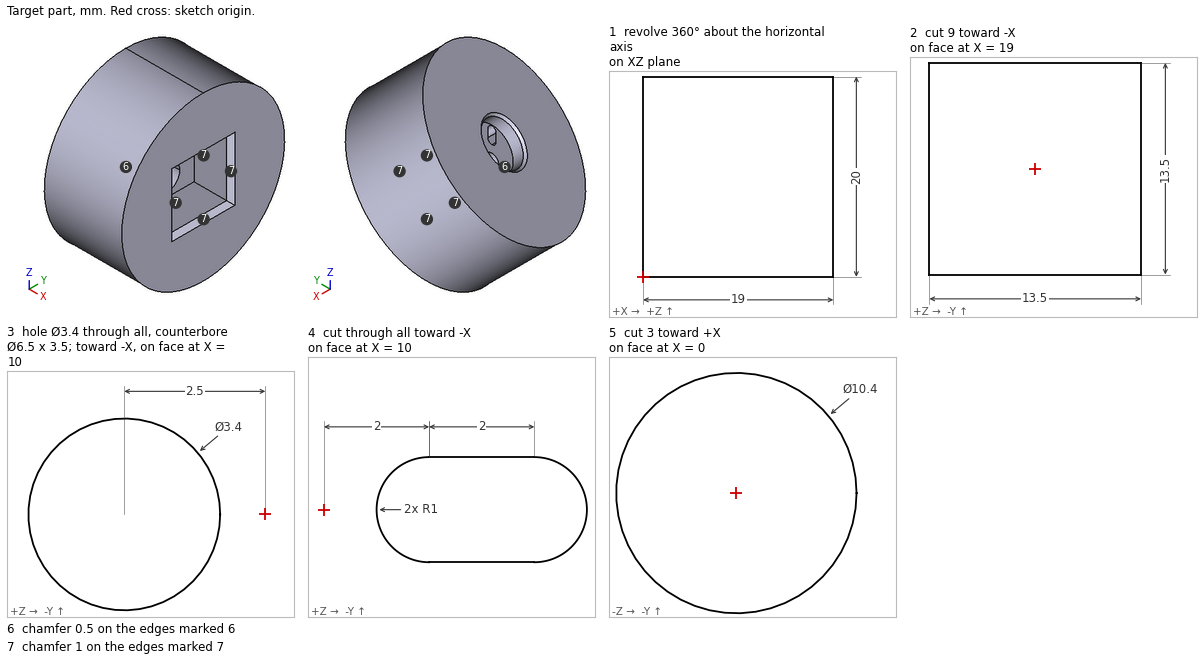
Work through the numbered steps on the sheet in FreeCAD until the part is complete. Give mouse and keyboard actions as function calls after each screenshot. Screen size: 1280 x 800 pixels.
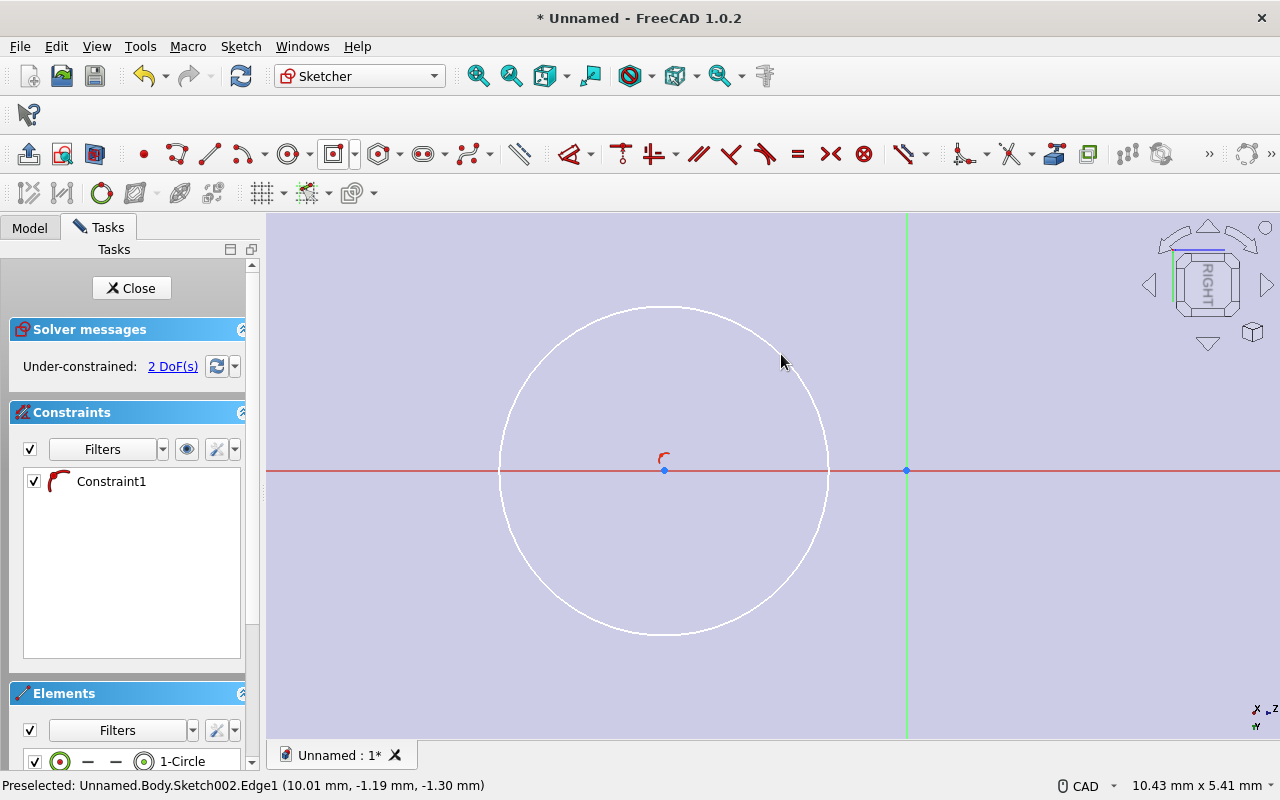
click(568, 154)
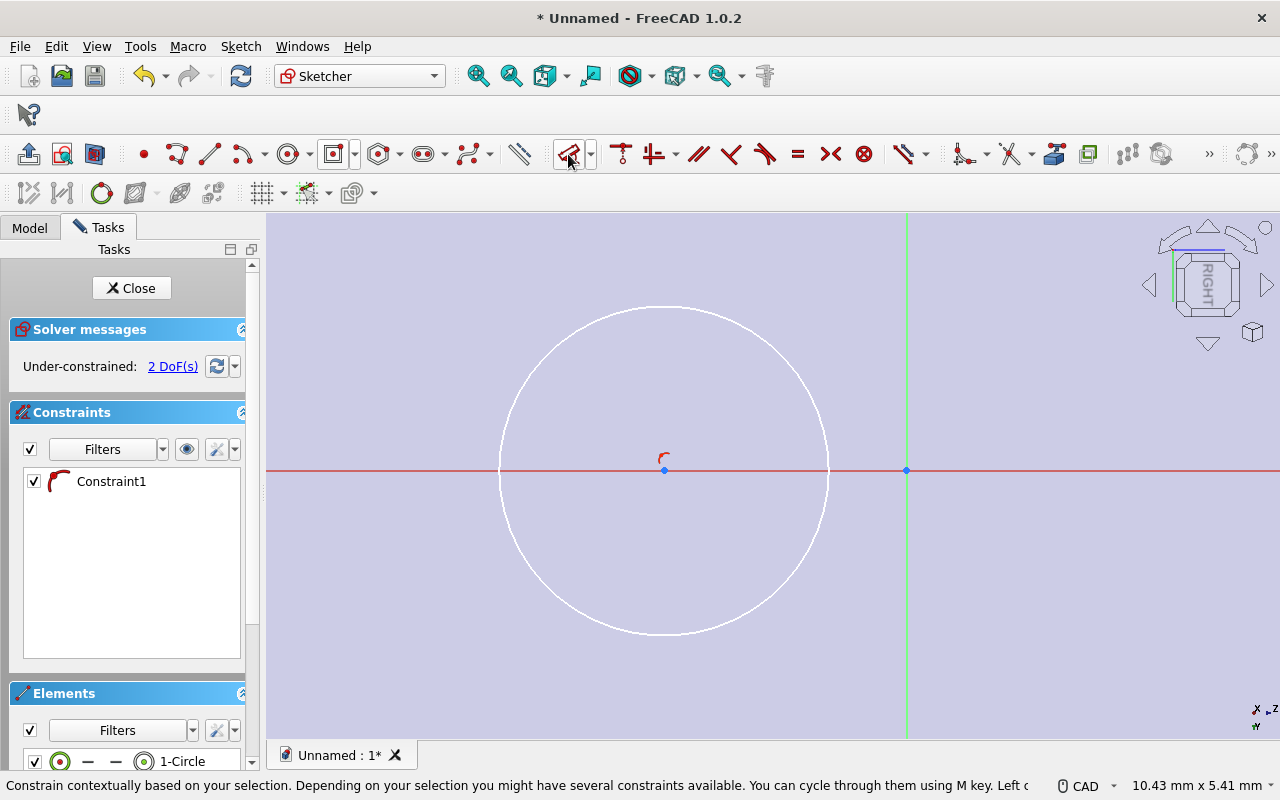
click(780, 354)
click(803, 331)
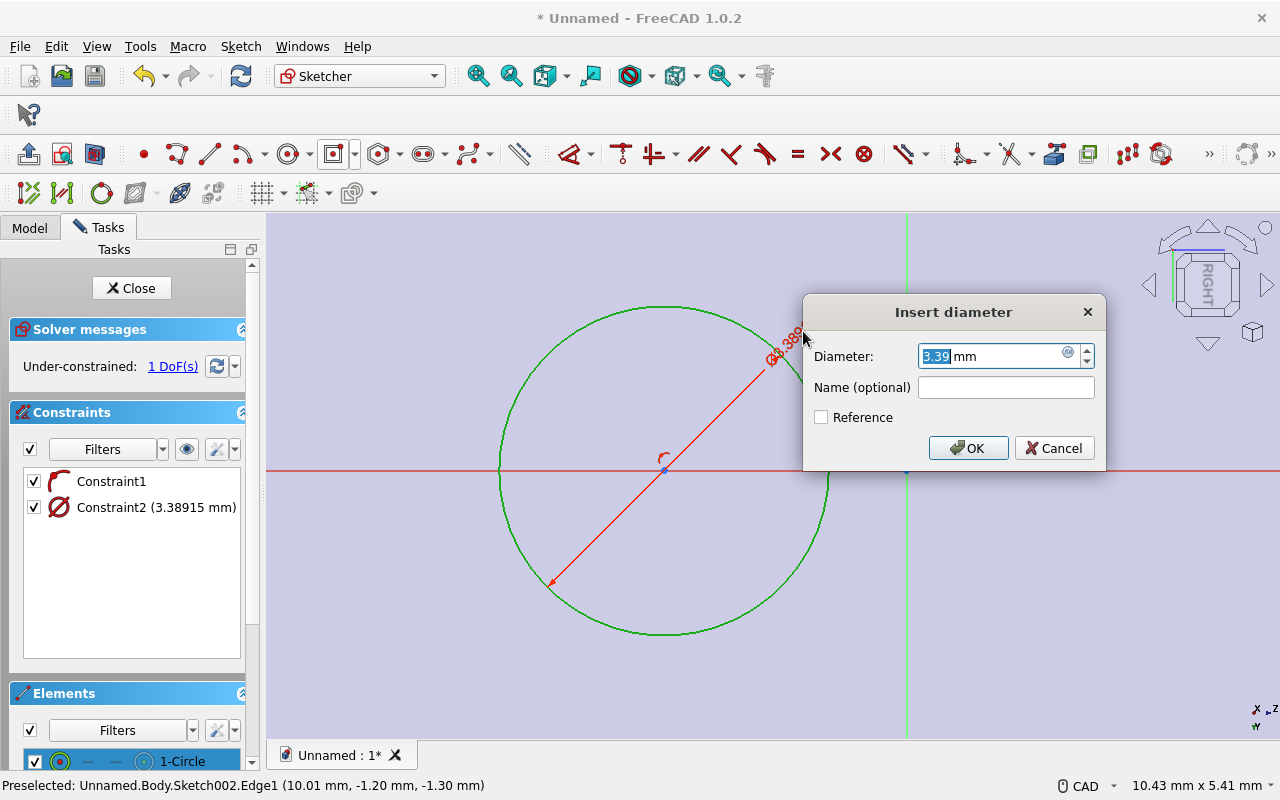
text(3.4)
key(Return)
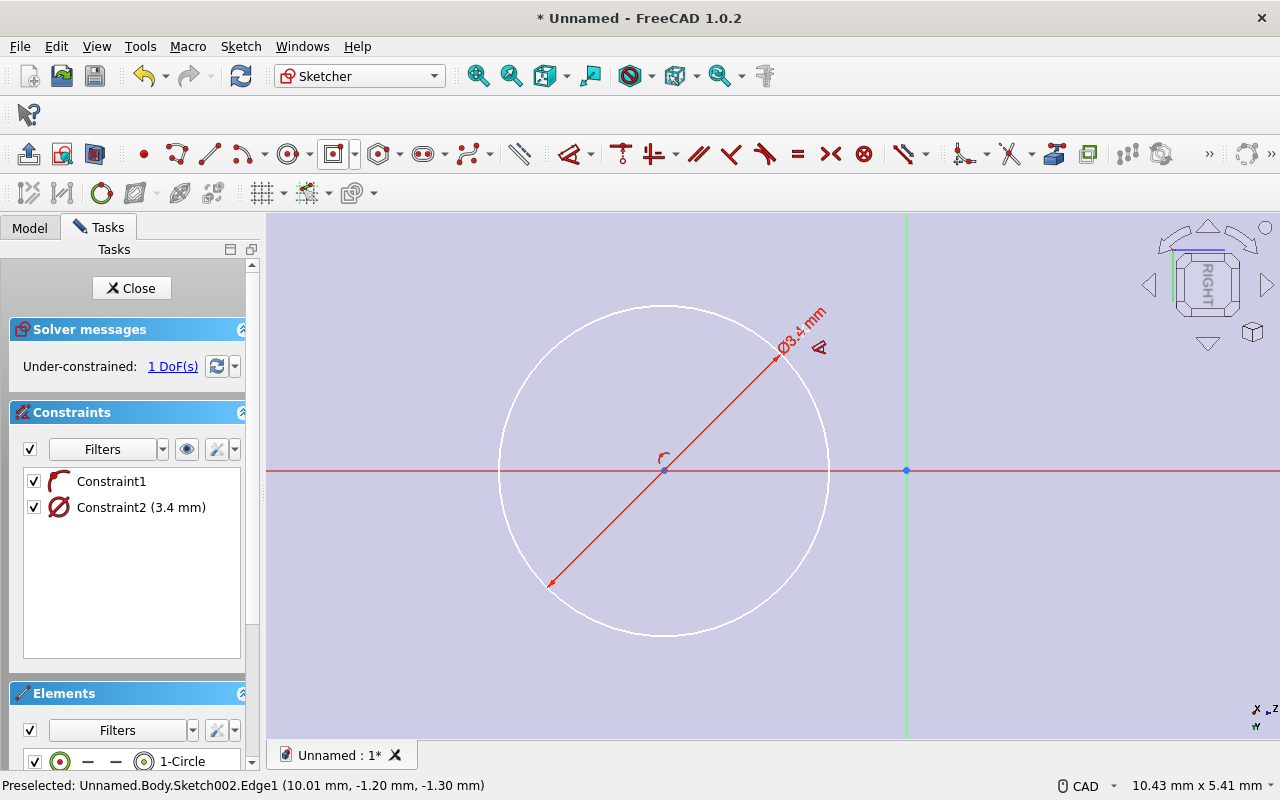
click(664, 471)
click(785, 505)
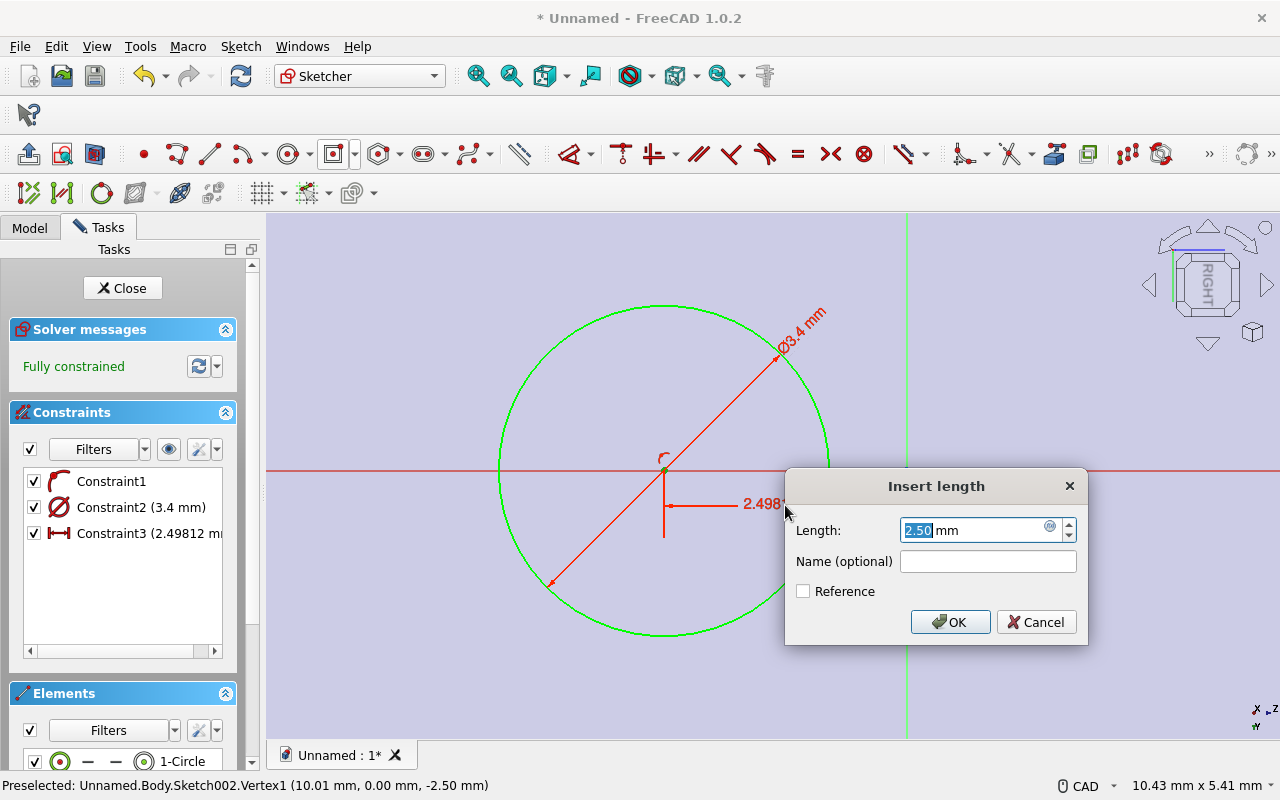
text(2.5)
key(Return)
key(Escape)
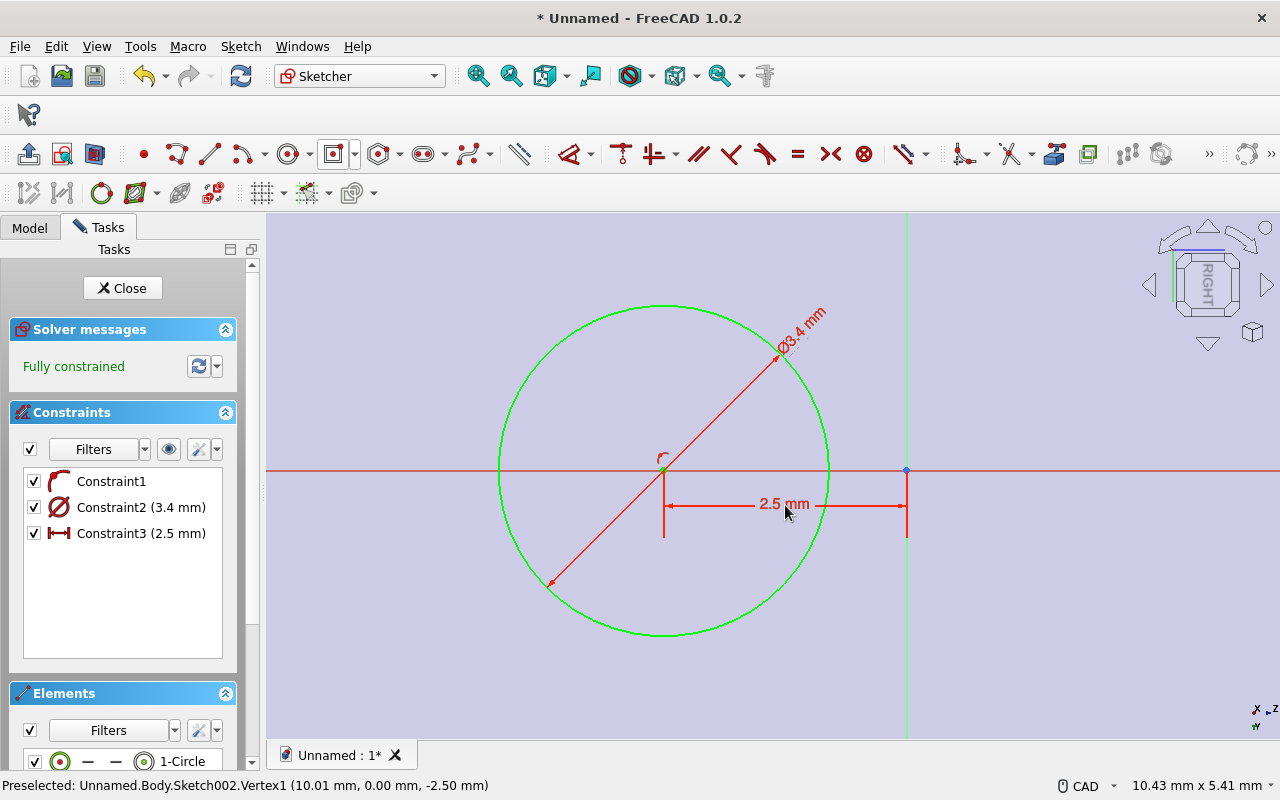
click(123, 288)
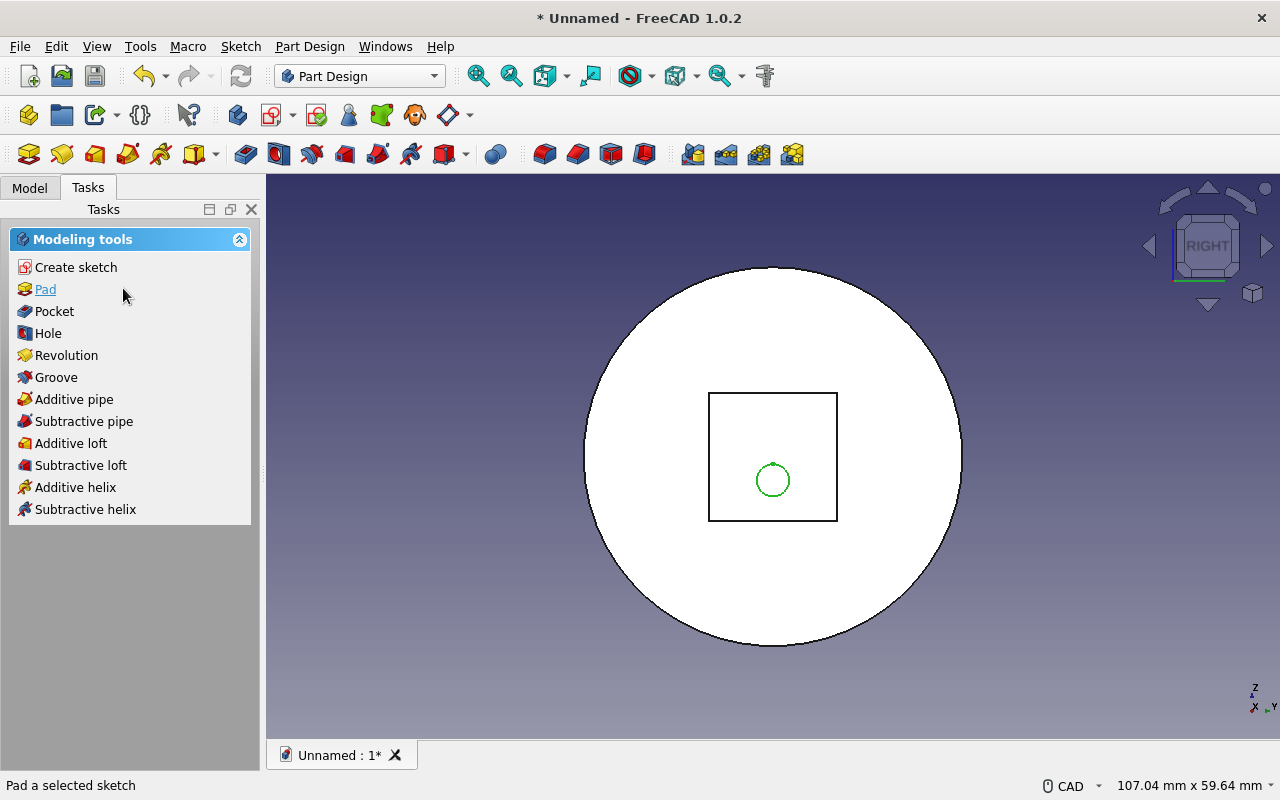
click(279, 154)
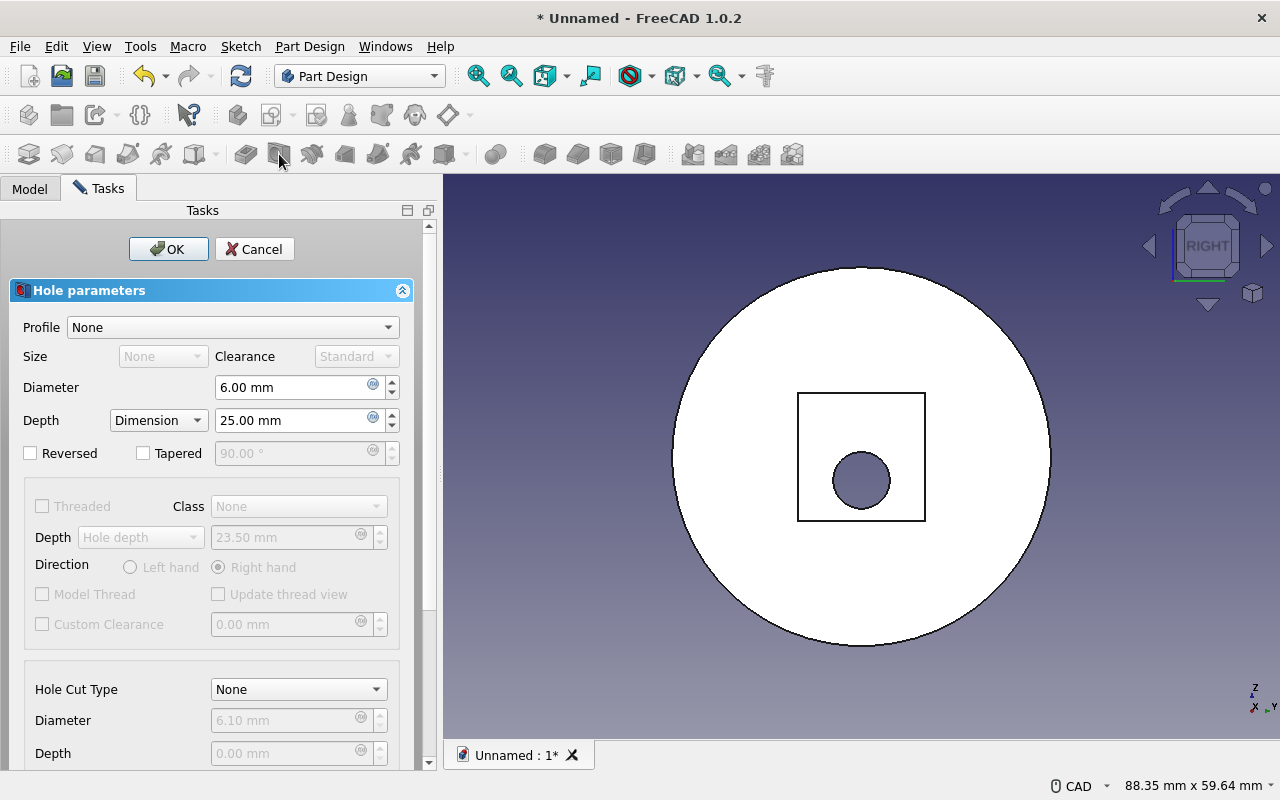
triple_click(300, 388)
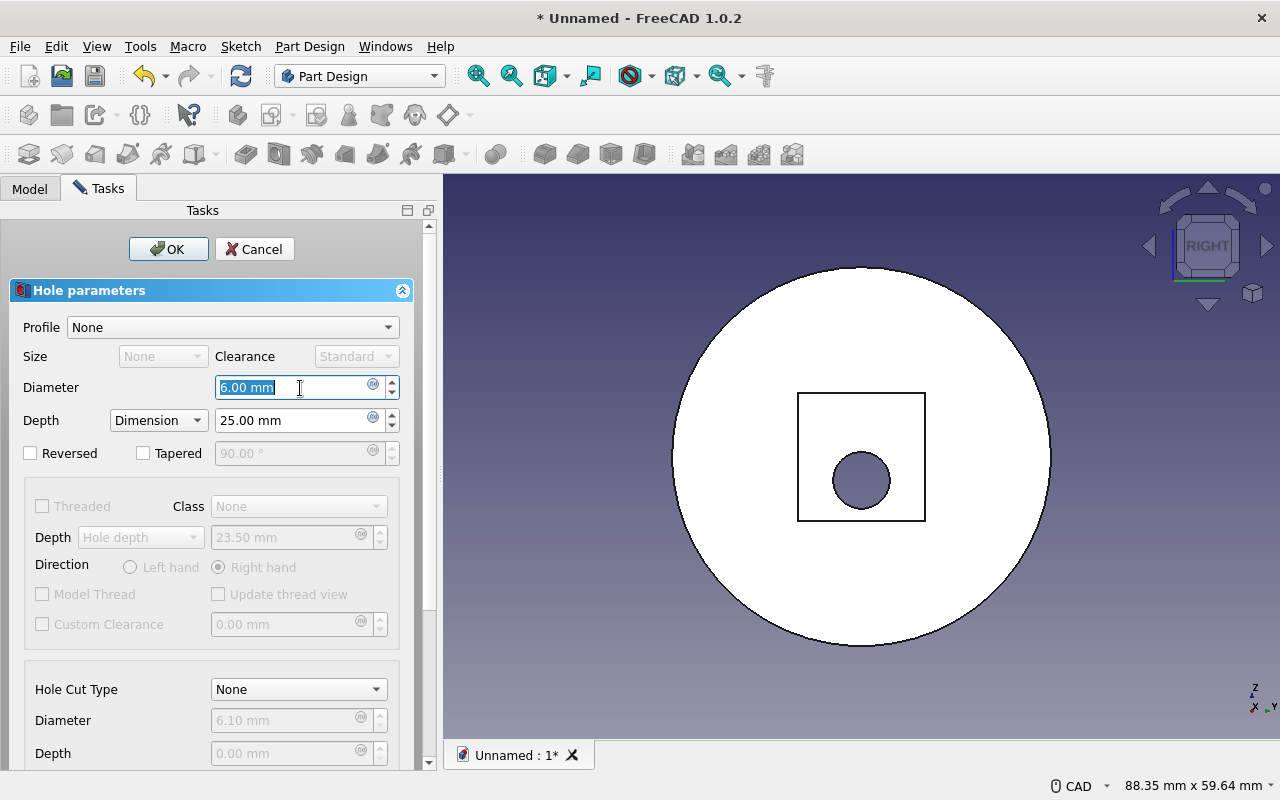
text(3.4)
key(Tab)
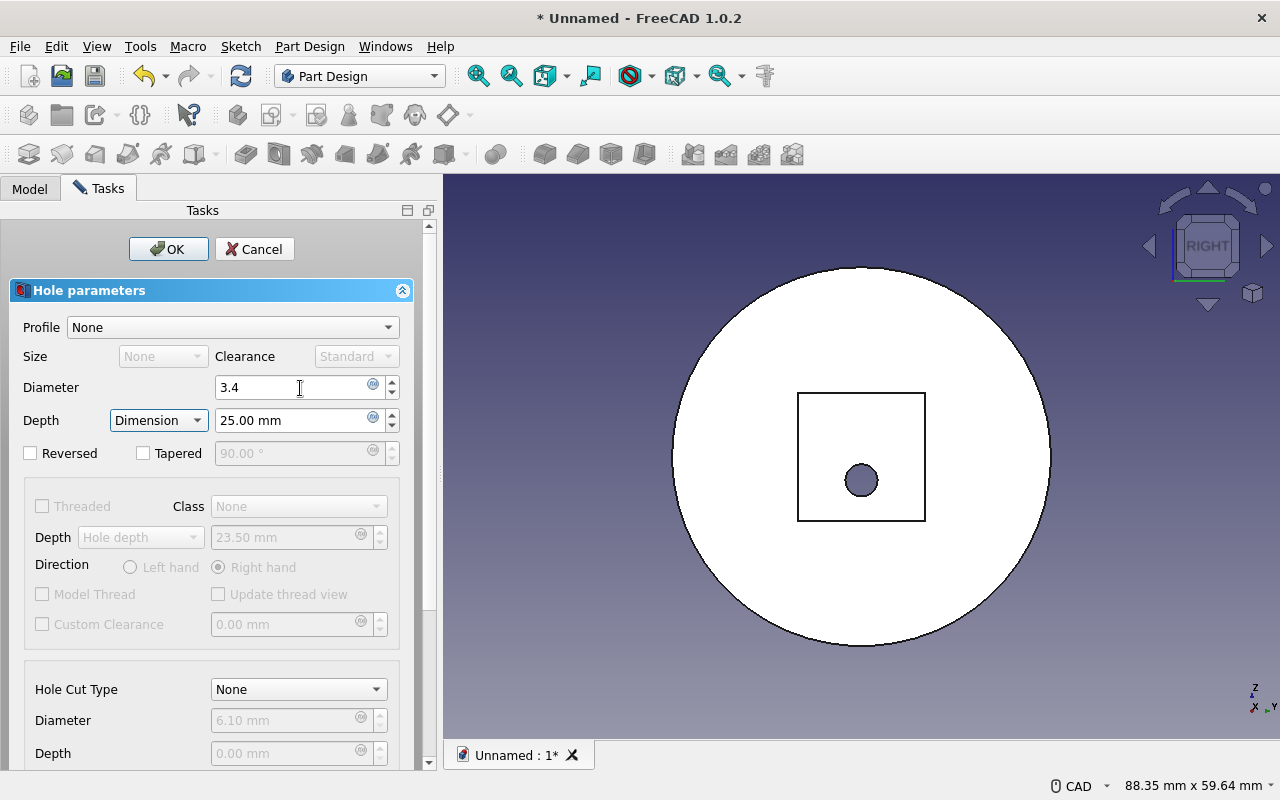
click(160, 420)